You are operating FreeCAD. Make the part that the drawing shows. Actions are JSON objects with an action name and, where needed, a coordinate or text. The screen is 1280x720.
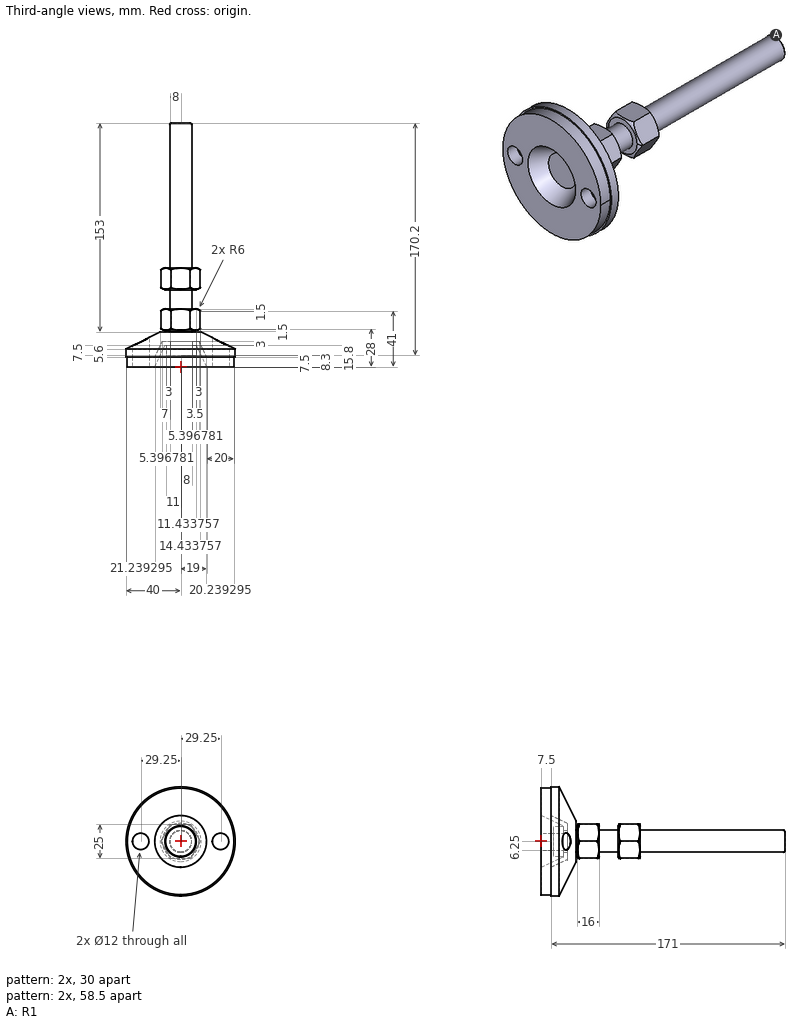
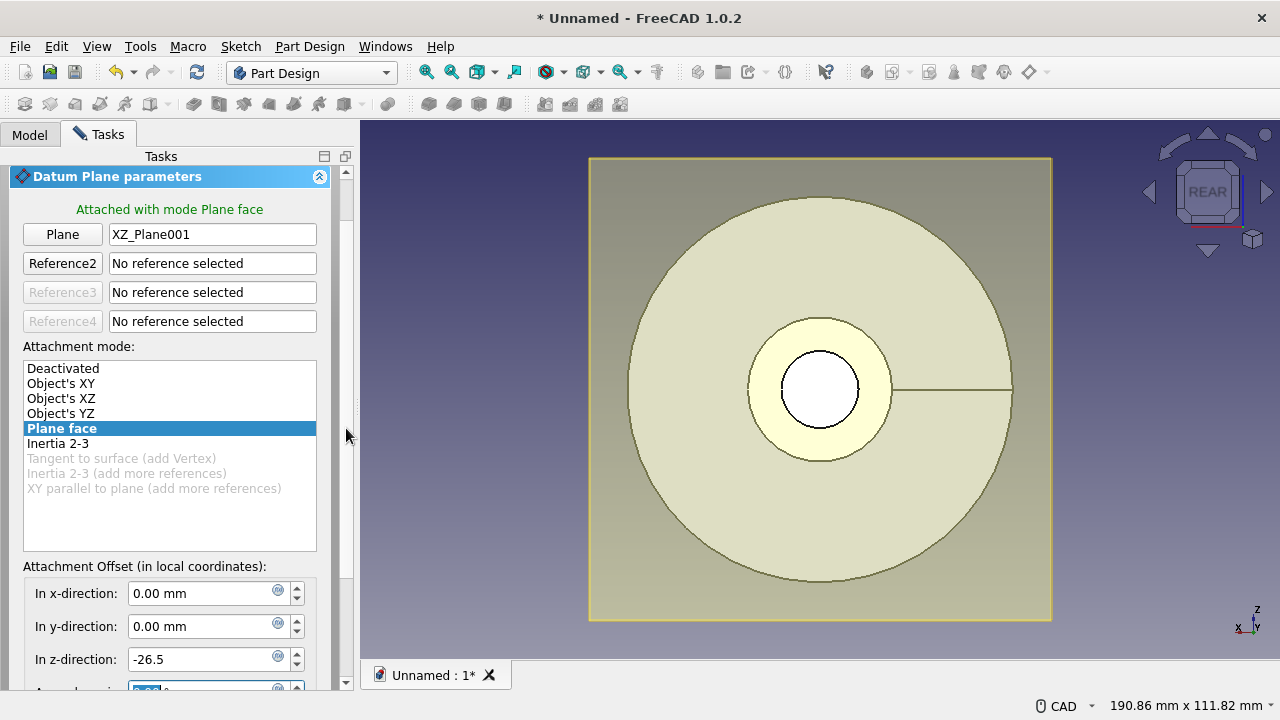
{"action": "left_click", "coordinate": [127, 195]}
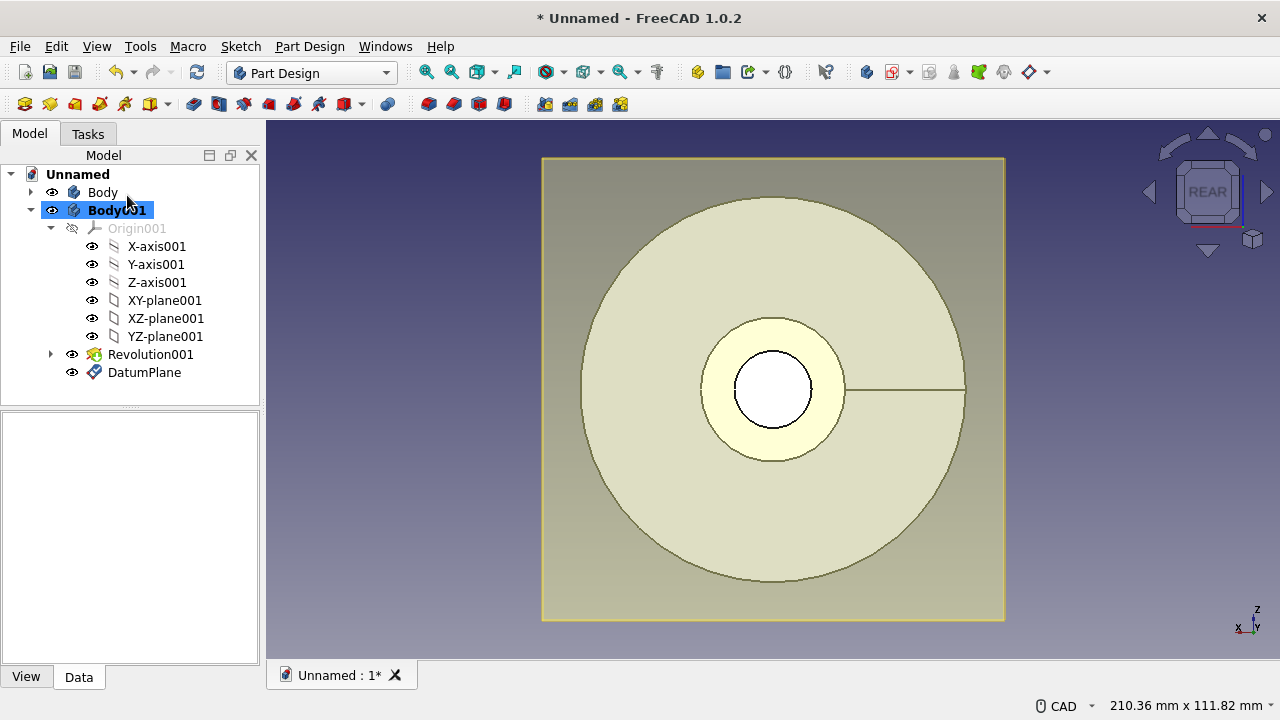
{"action": "left_click", "coordinate": [117, 372]}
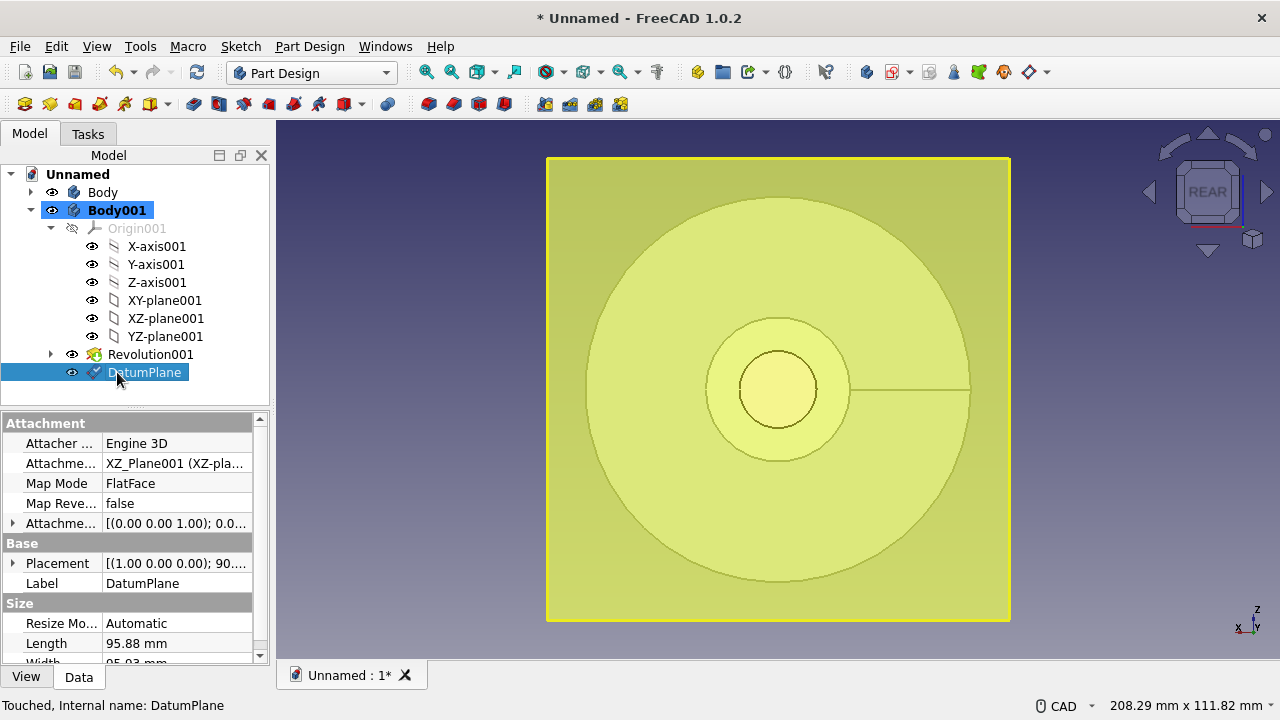
{"action": "left_click", "coordinate": [892, 72]}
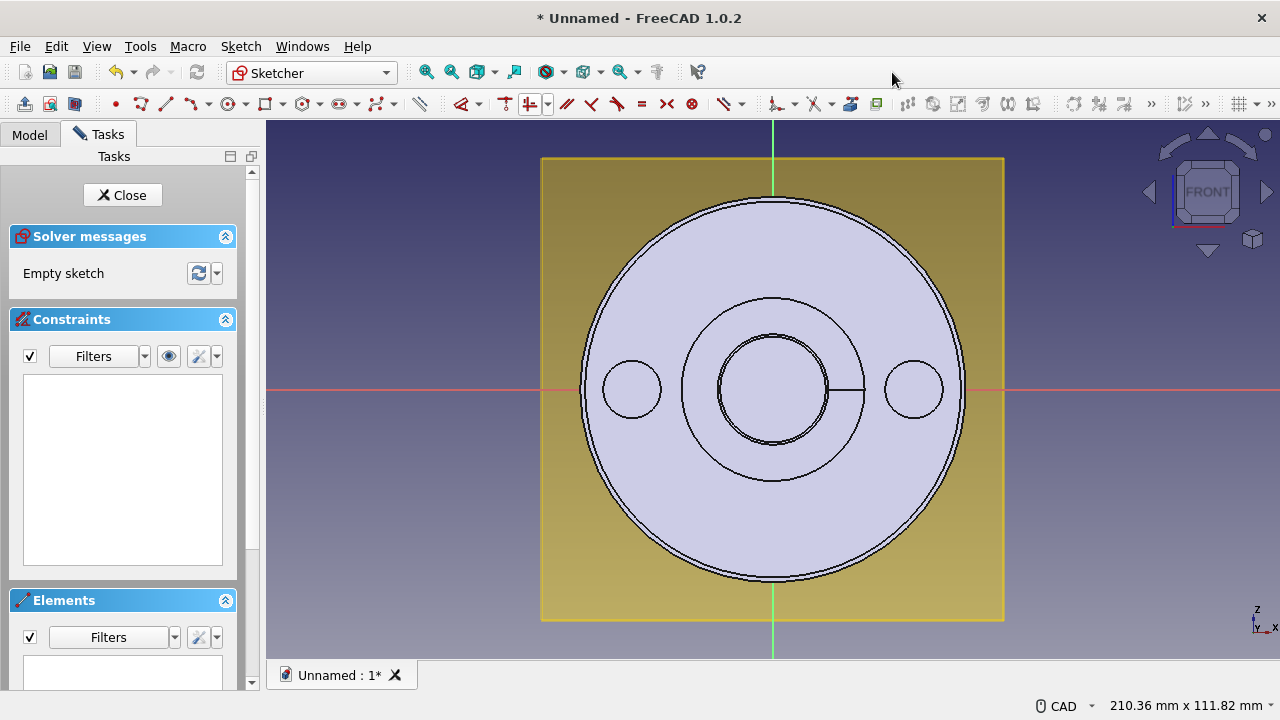
{"action": "left_click", "coordinate": [75, 104]}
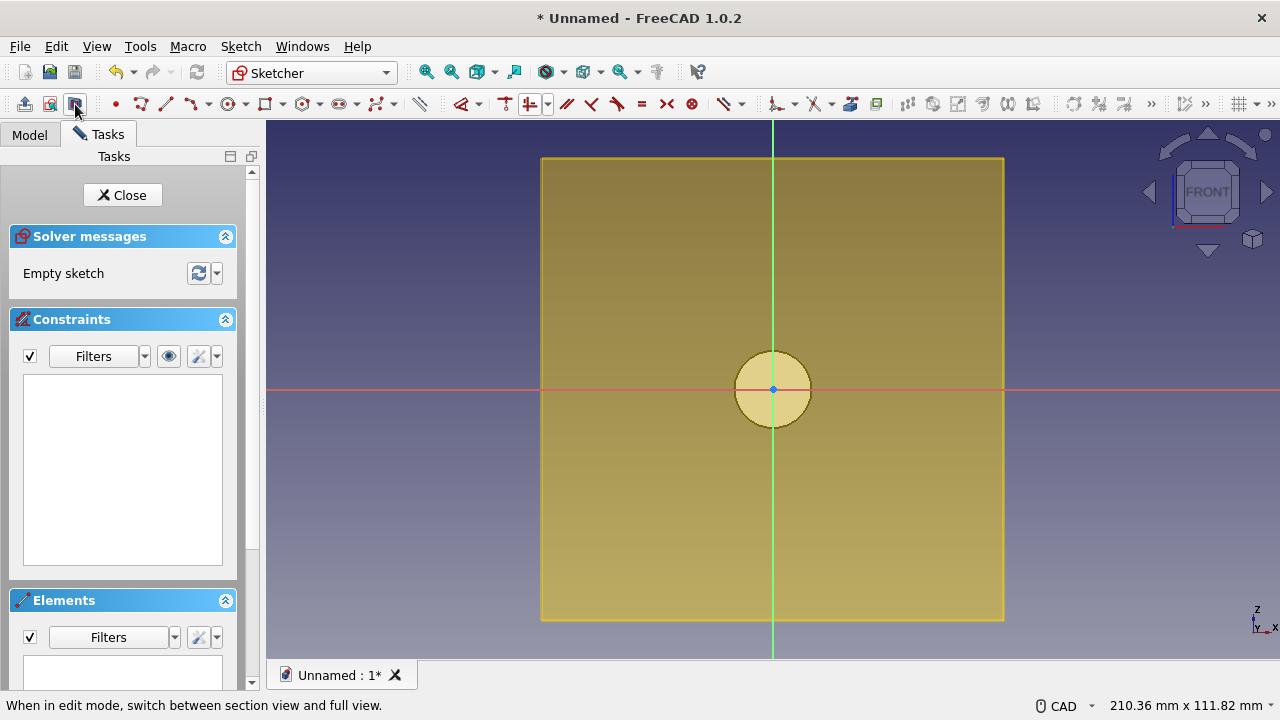
{"action": "scroll", "coordinate": [813, 390], "scroll_direction": "up", "scroll_amount": 5}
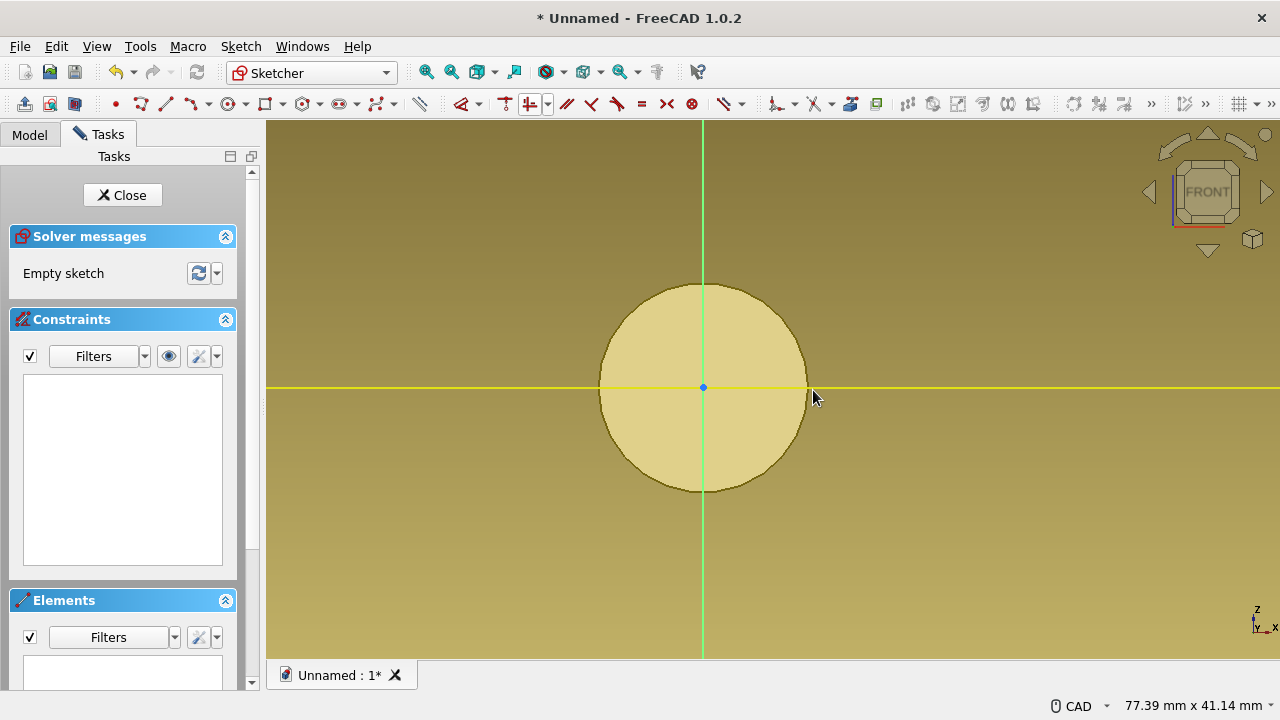
{"action": "left_click", "coordinate": [302, 104]}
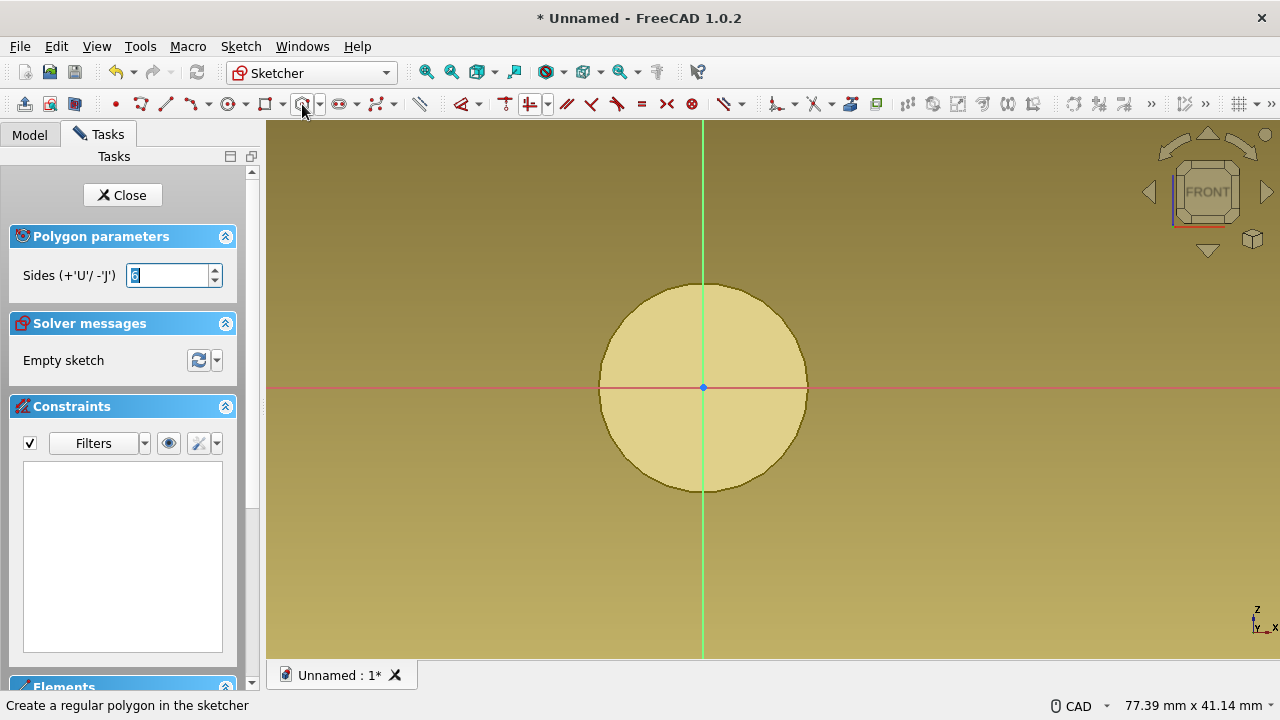
{"action": "left_click", "coordinate": [703, 388]}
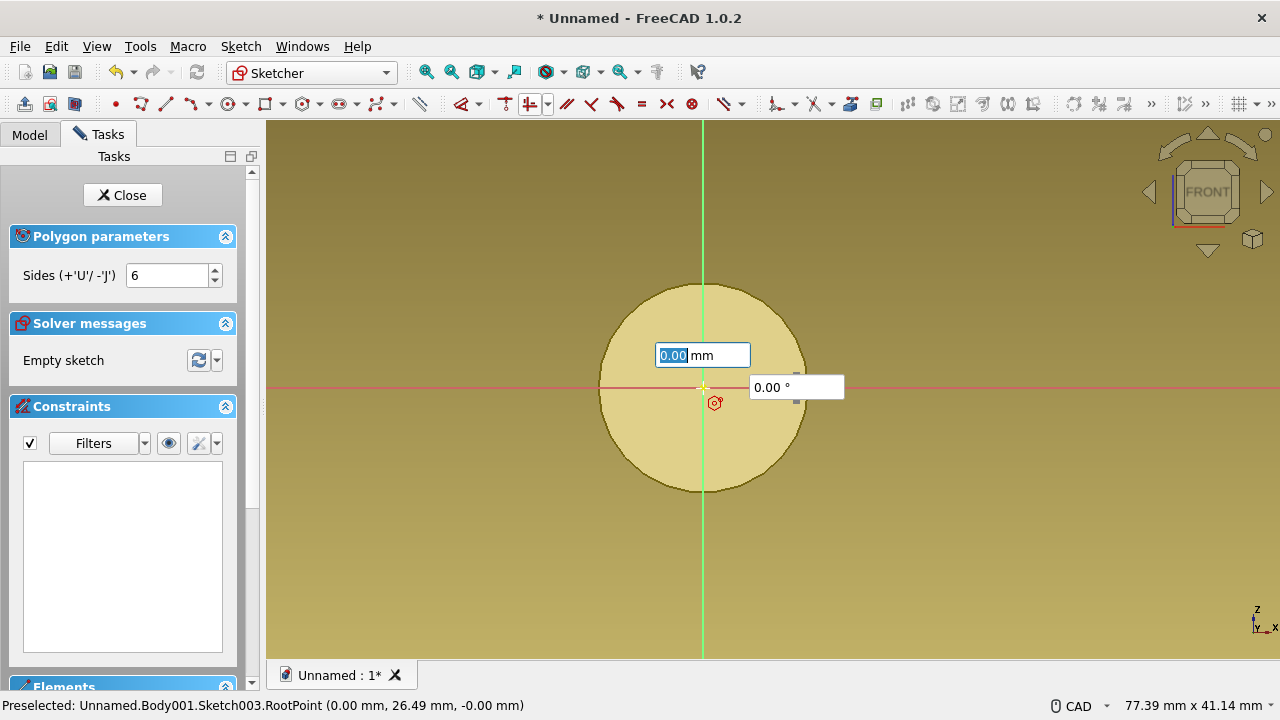
{"action": "left_click", "coordinate": [892, 388]}
{"action": "right_click", "coordinate": [892, 388]}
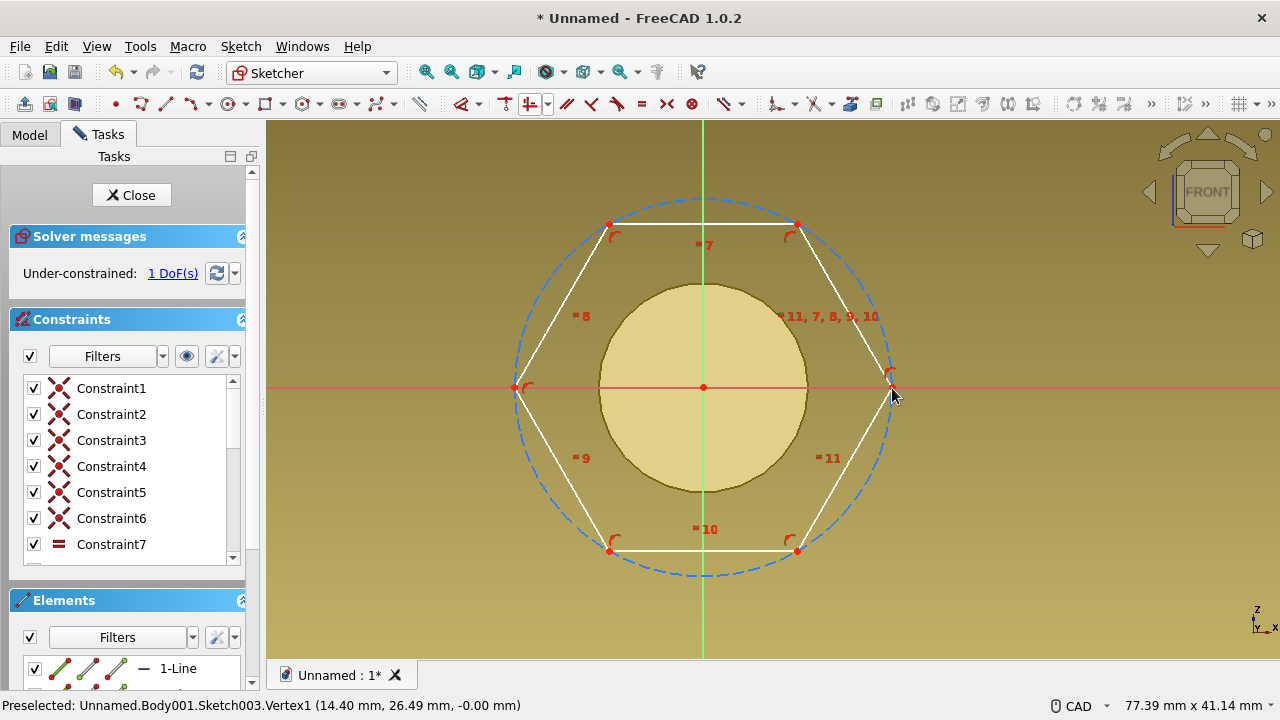
{"action": "left_click", "coordinate": [460, 104]}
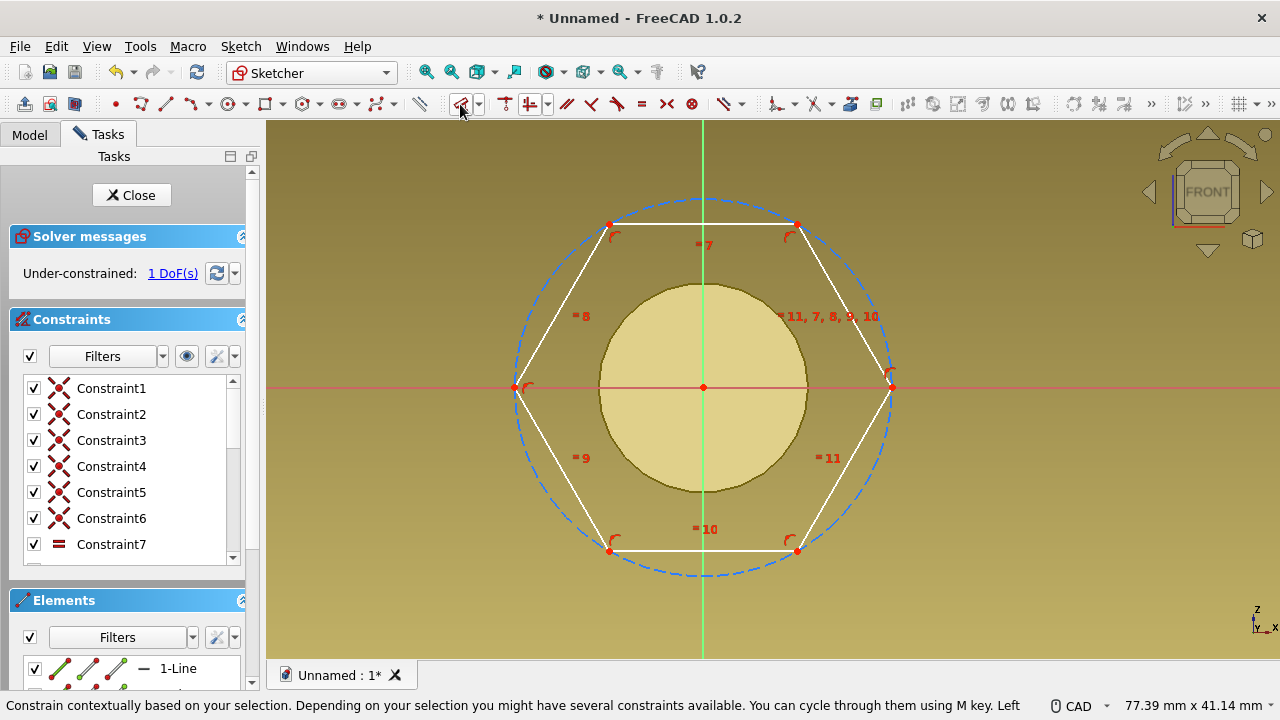
{"action": "left_click", "coordinate": [609, 551]}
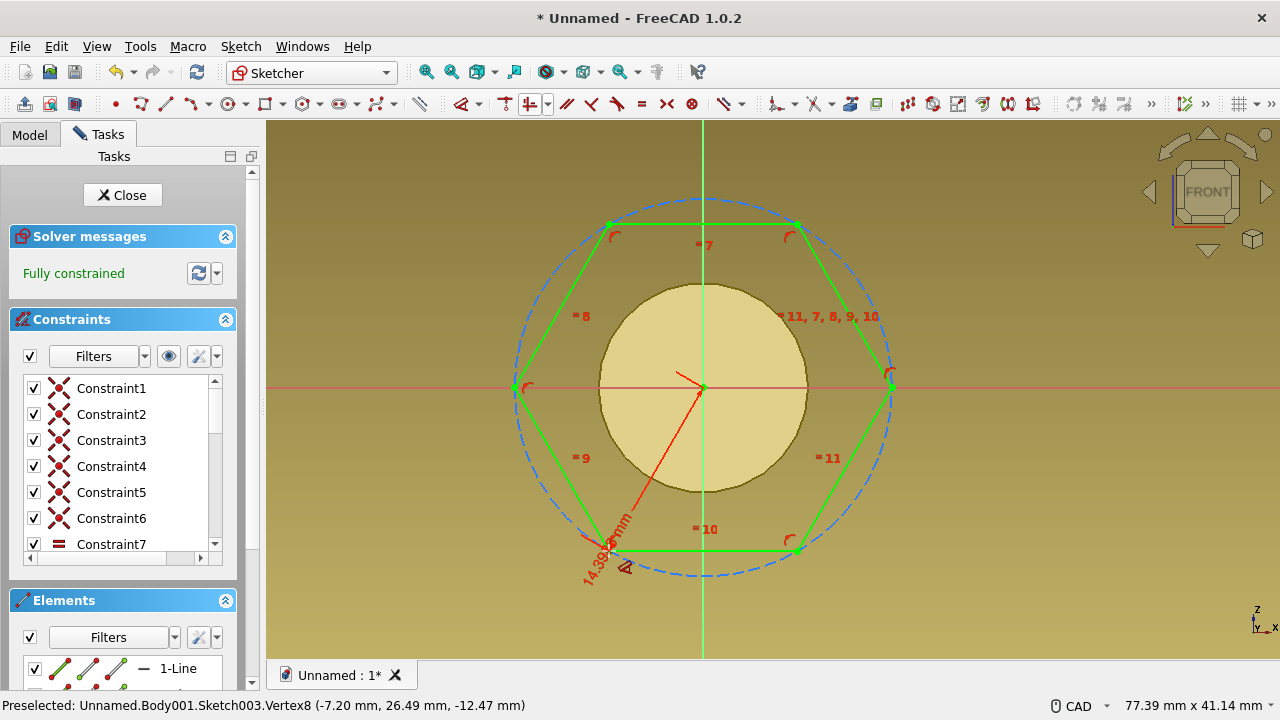
{"action": "left_click", "coordinate": [798, 224]}
{"action": "left_click", "coordinate": [832, 313]}